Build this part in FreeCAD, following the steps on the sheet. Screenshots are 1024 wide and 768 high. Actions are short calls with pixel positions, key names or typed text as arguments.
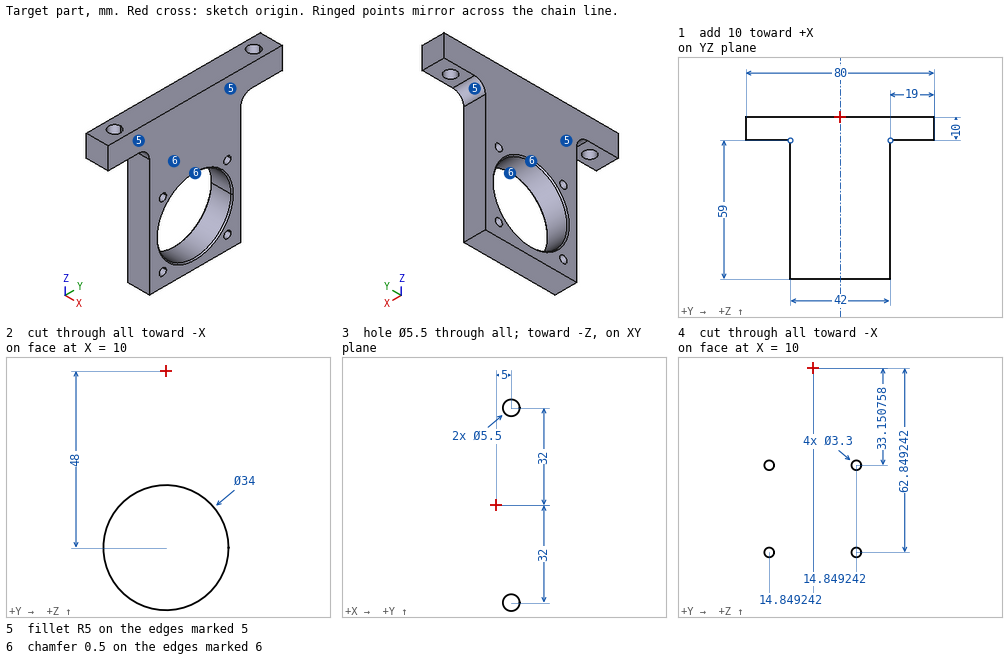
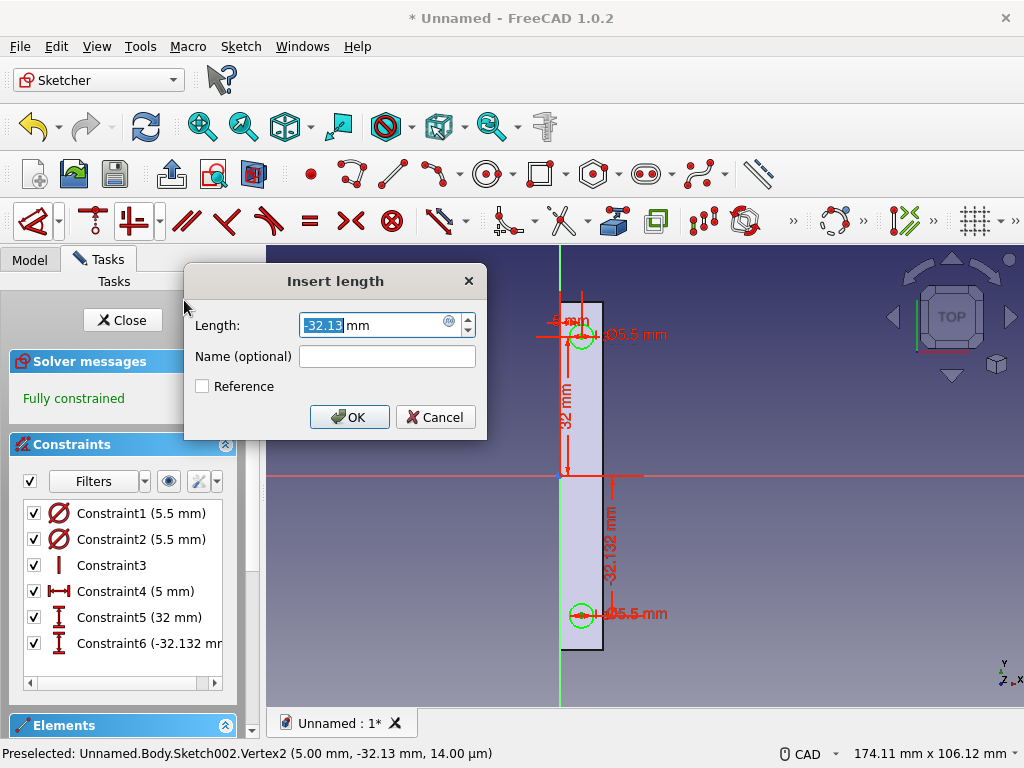
text(-32)
key(Return)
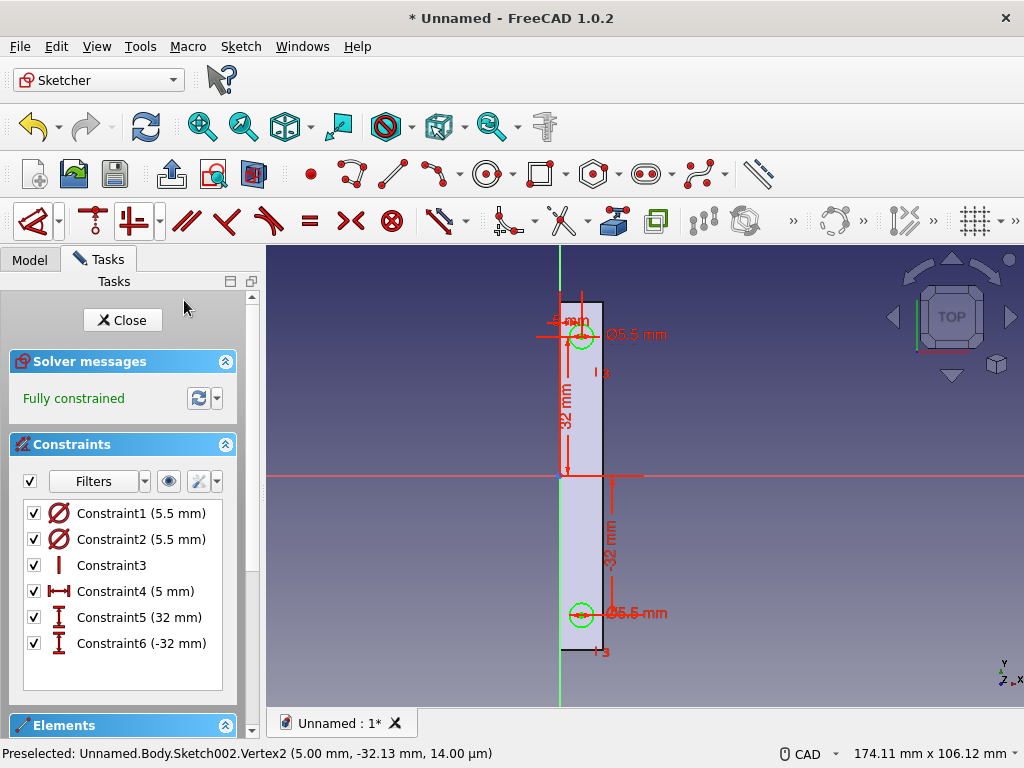
click(123, 320)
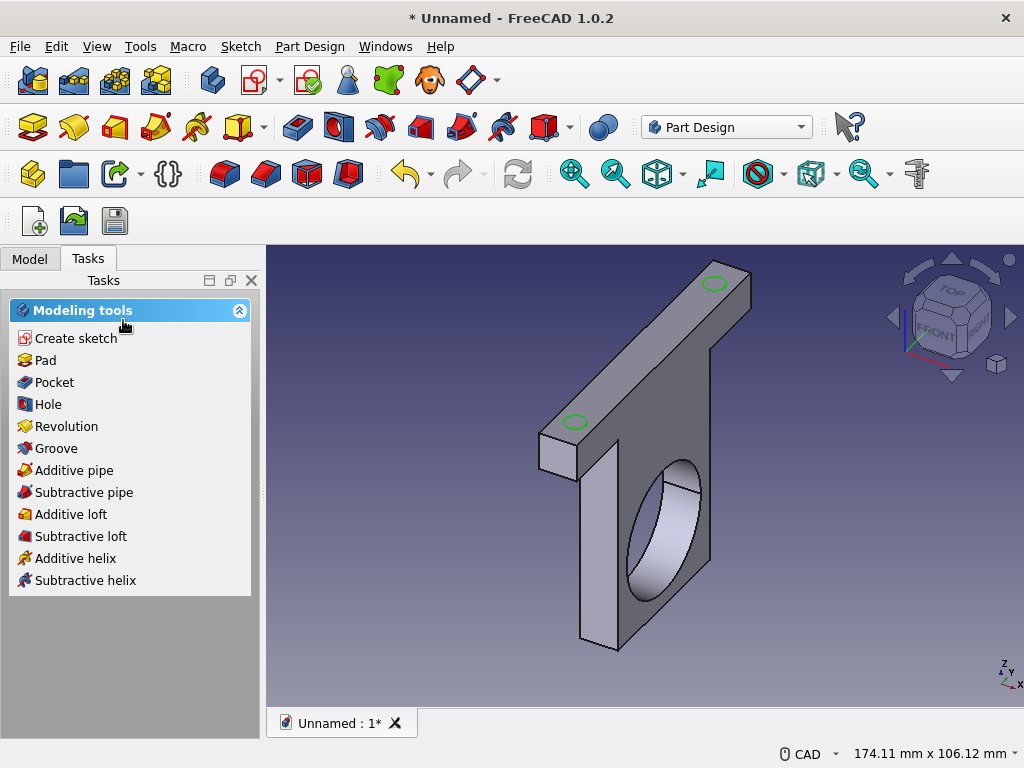
click(339, 128)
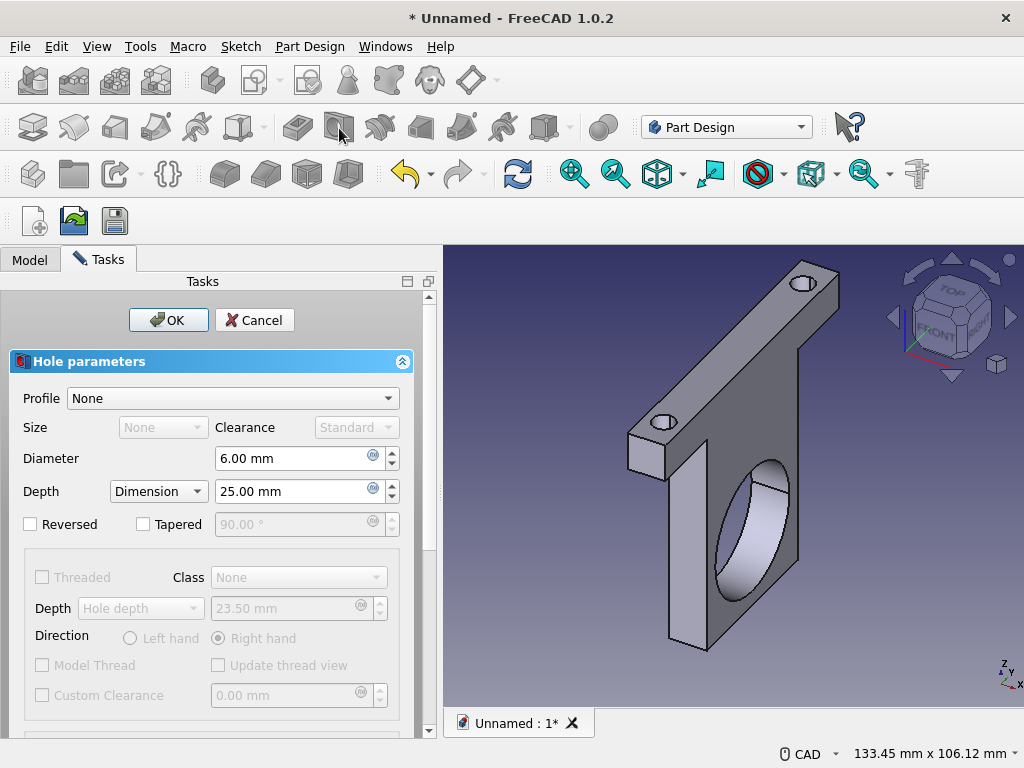
triple_click(300, 458)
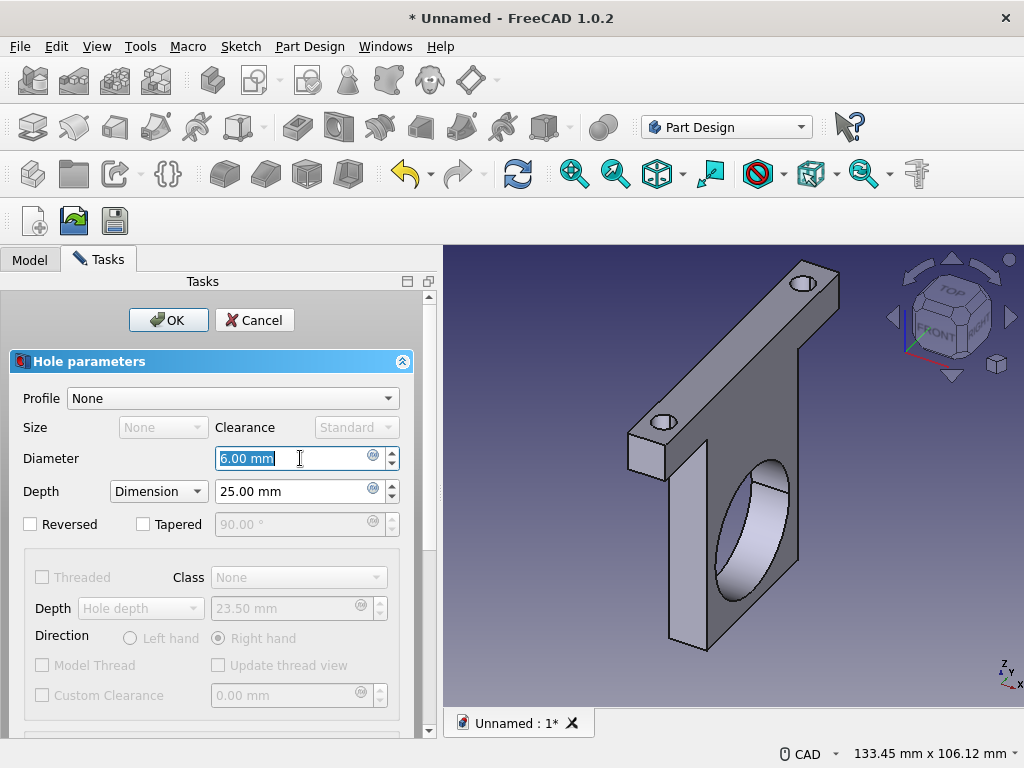
text(5.5)
key(Tab)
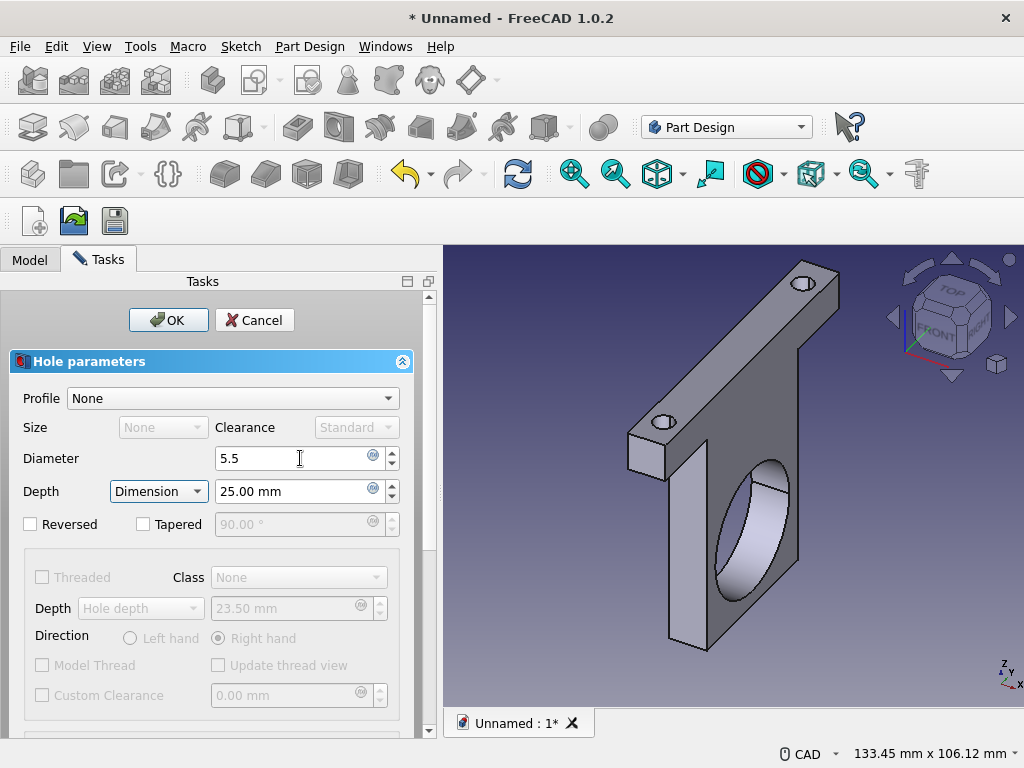
click(160, 492)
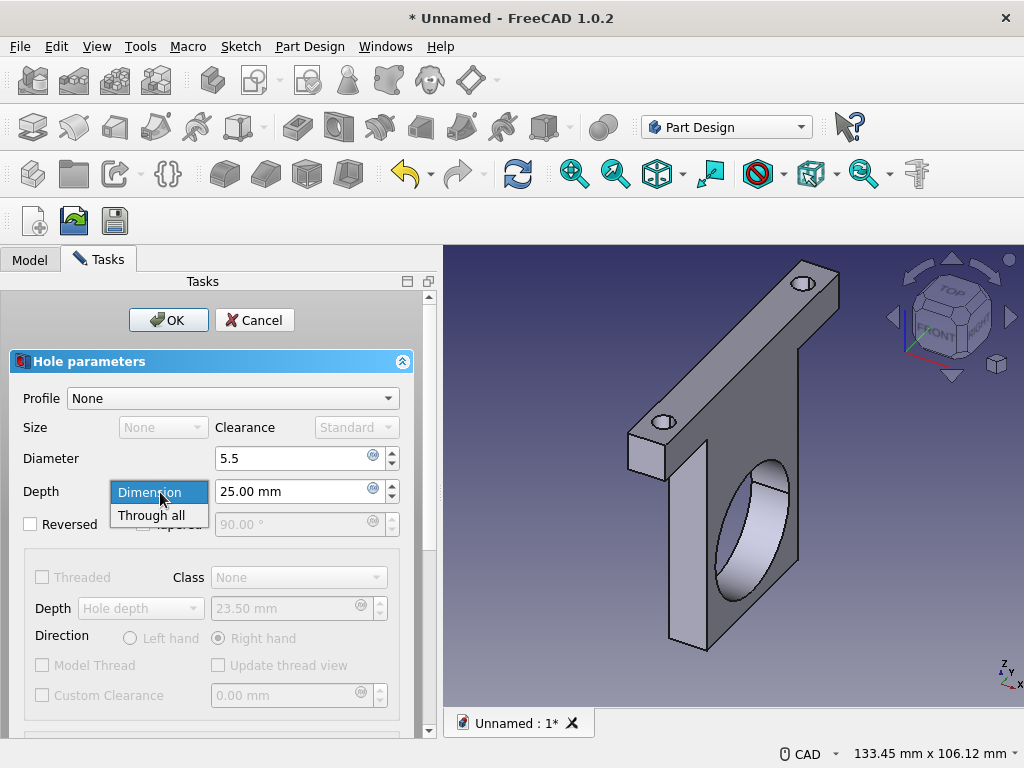
click(158, 516)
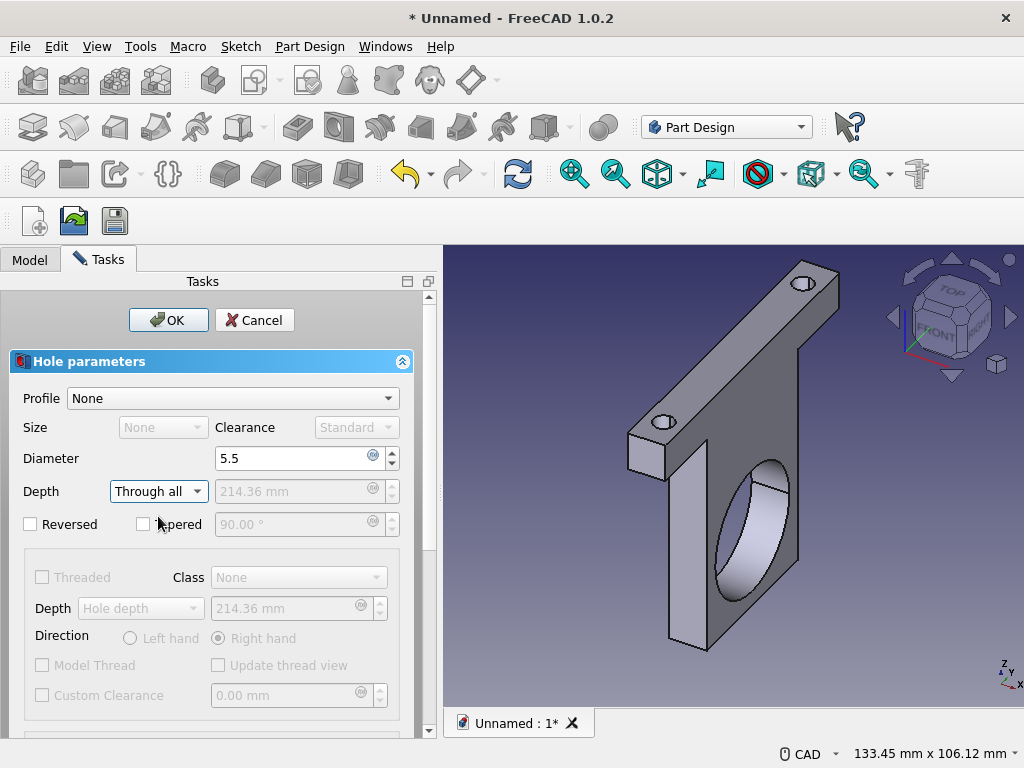
click(169, 320)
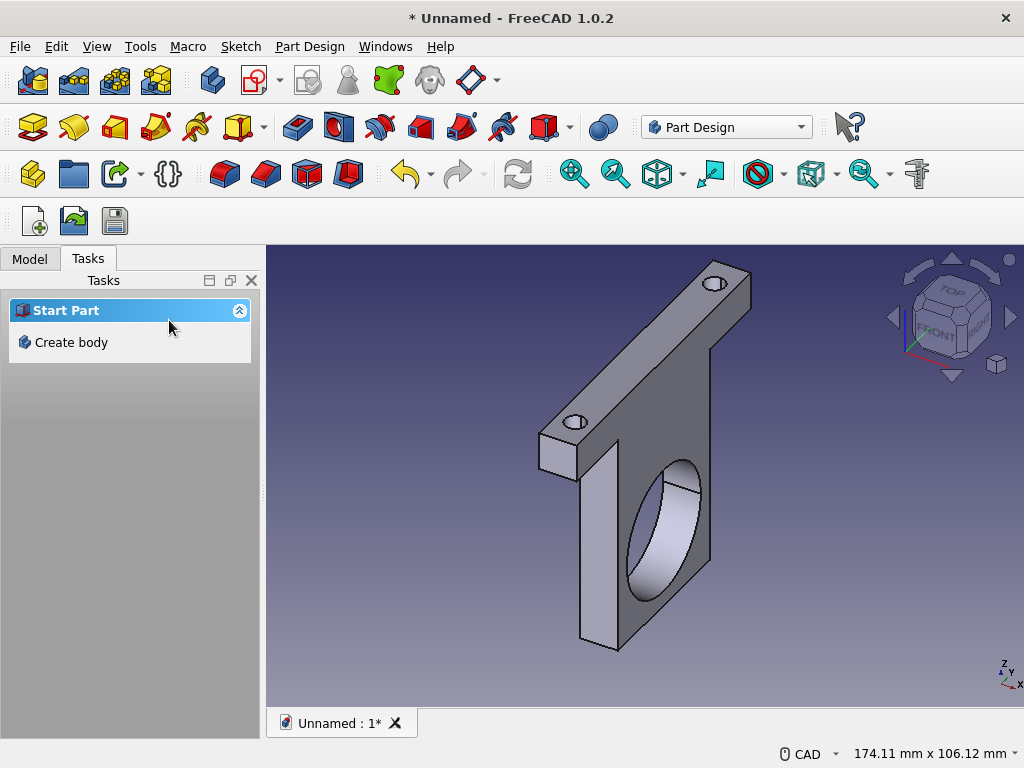
click(664, 411)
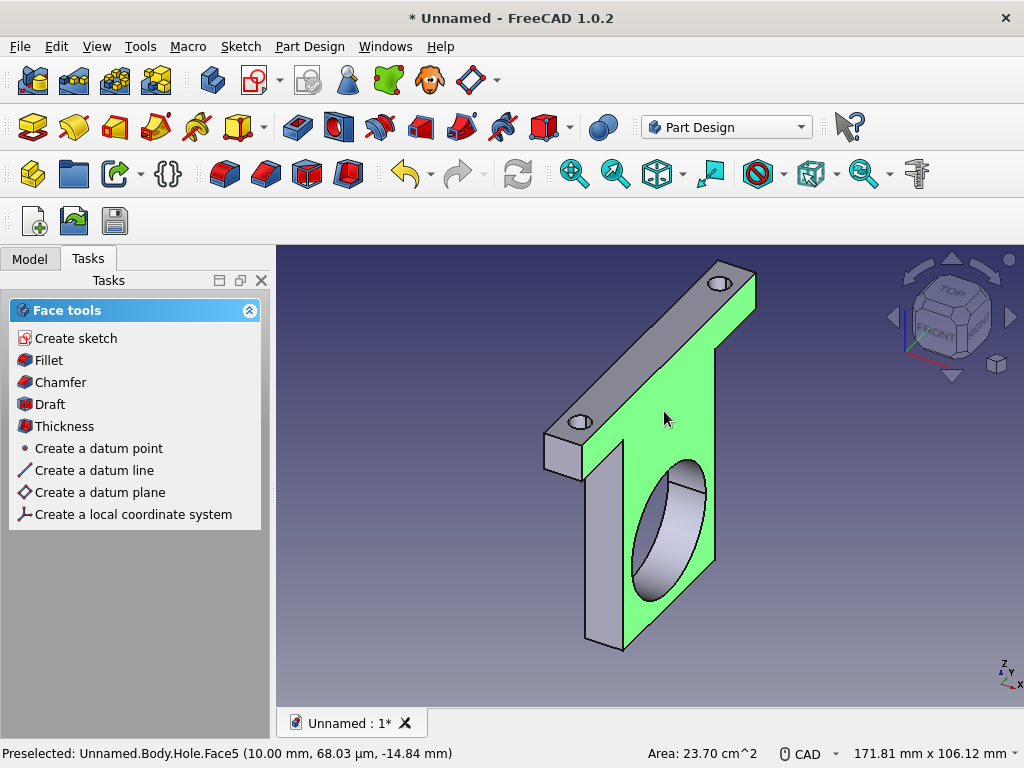
click(254, 80)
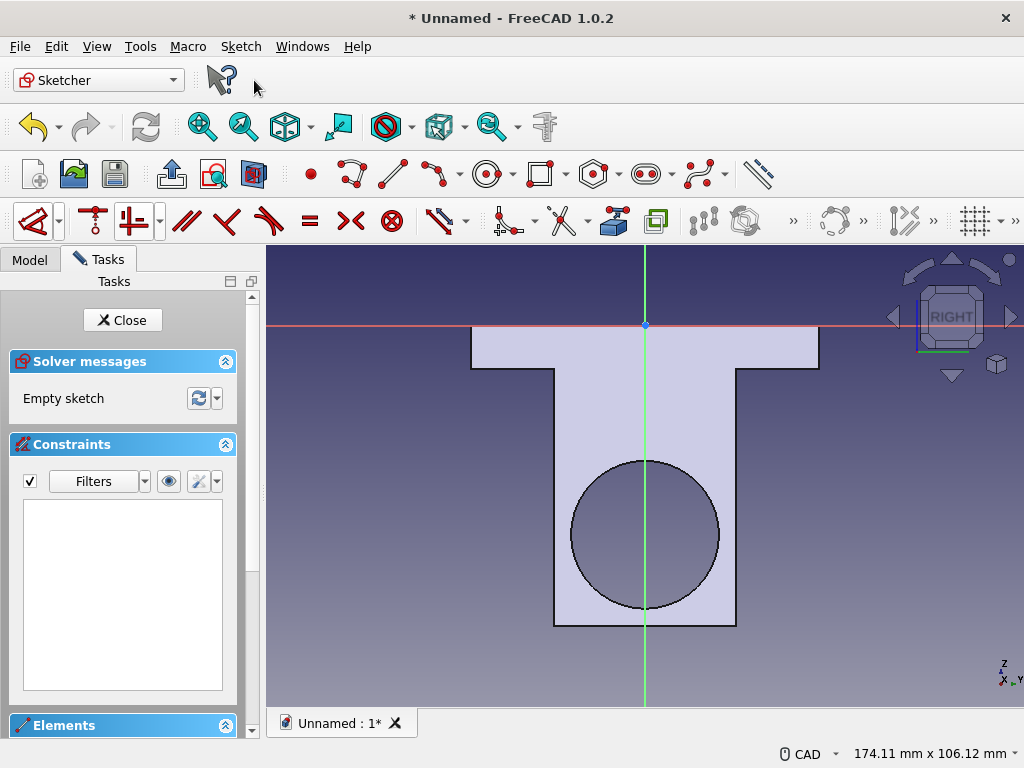
click(486, 174)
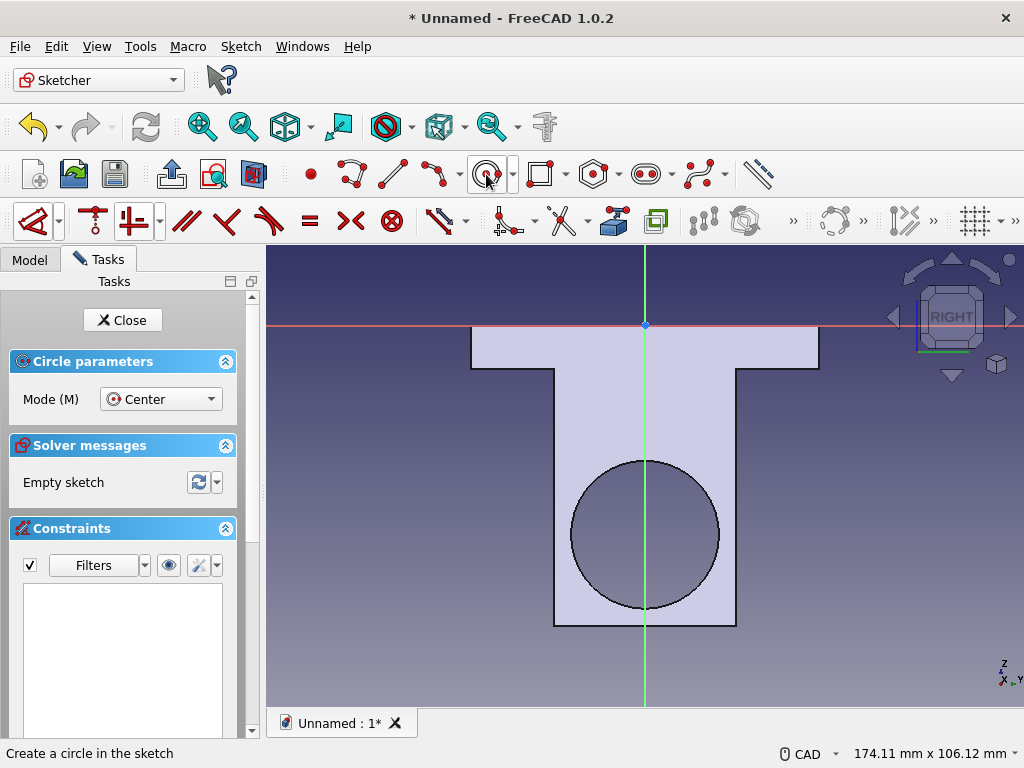
scroll(710, 470, up, 6)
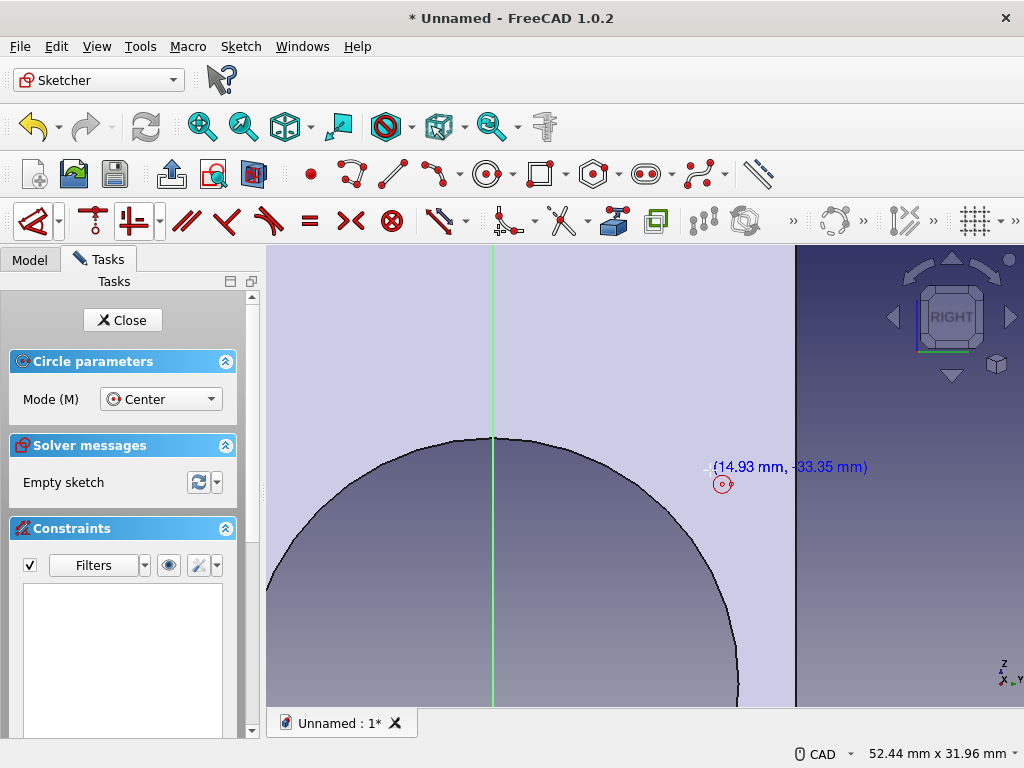
click(707, 469)
move(724, 452)